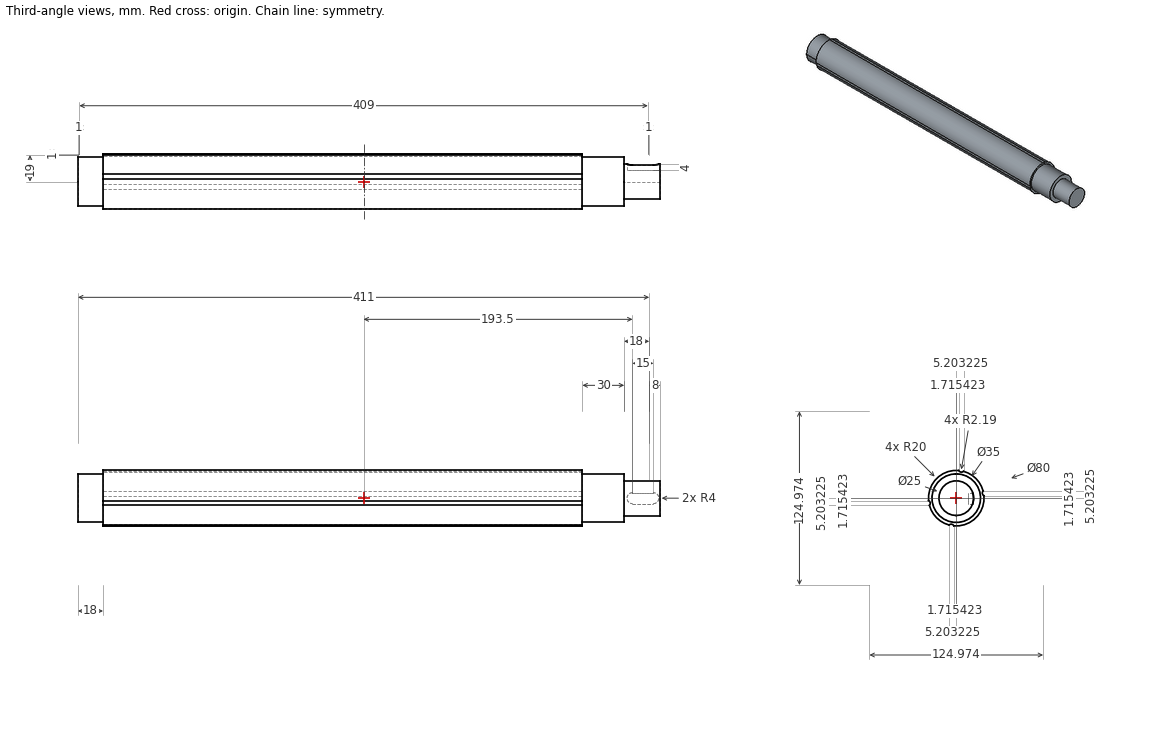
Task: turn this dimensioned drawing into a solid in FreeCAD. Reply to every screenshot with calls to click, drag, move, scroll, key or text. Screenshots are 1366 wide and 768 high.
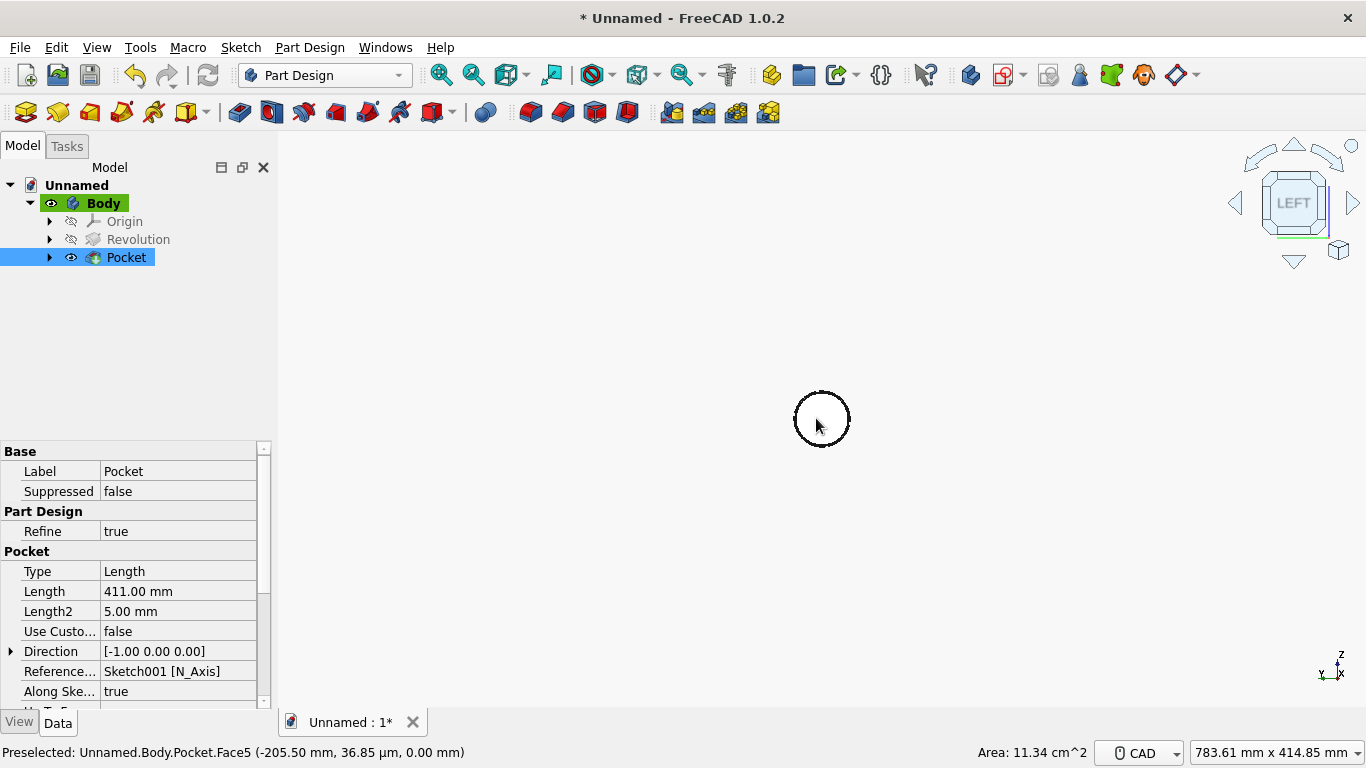
click(1004, 76)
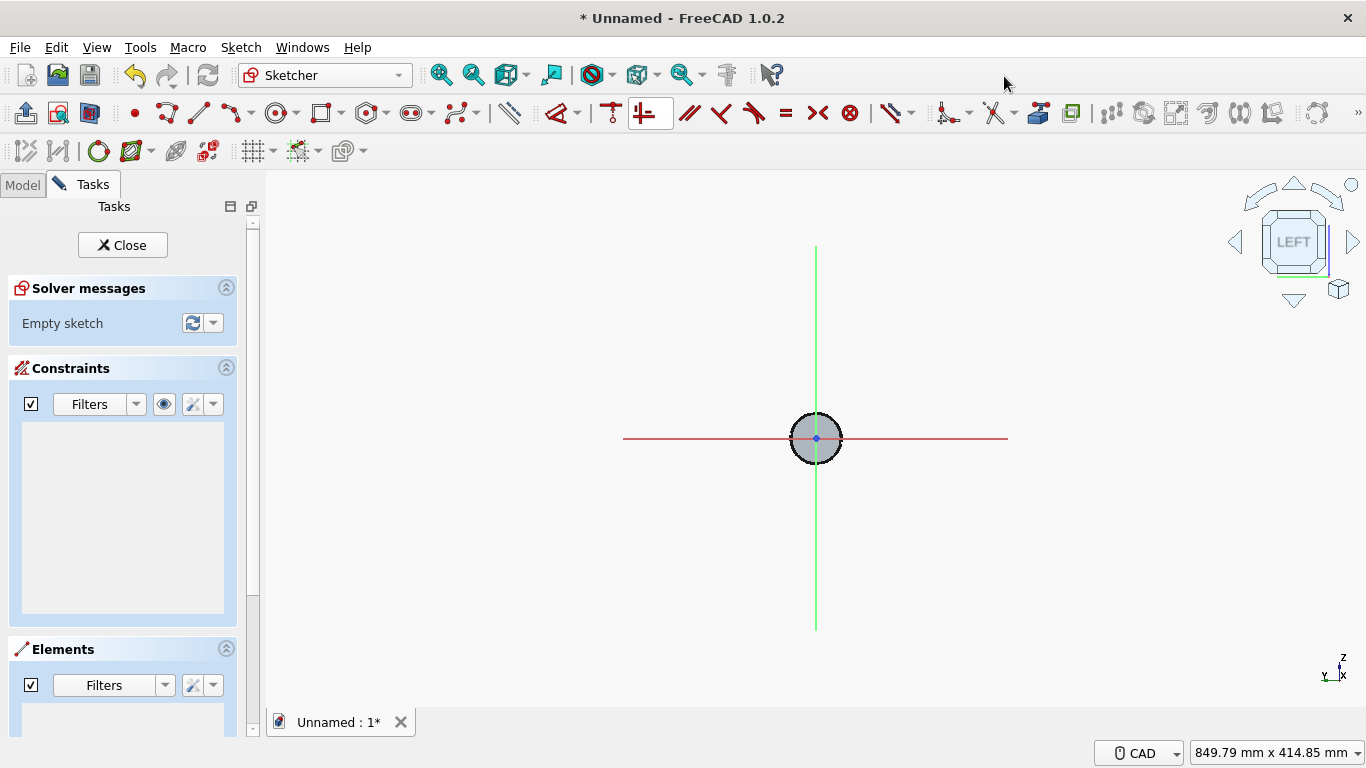
scroll(872, 438, up, 4)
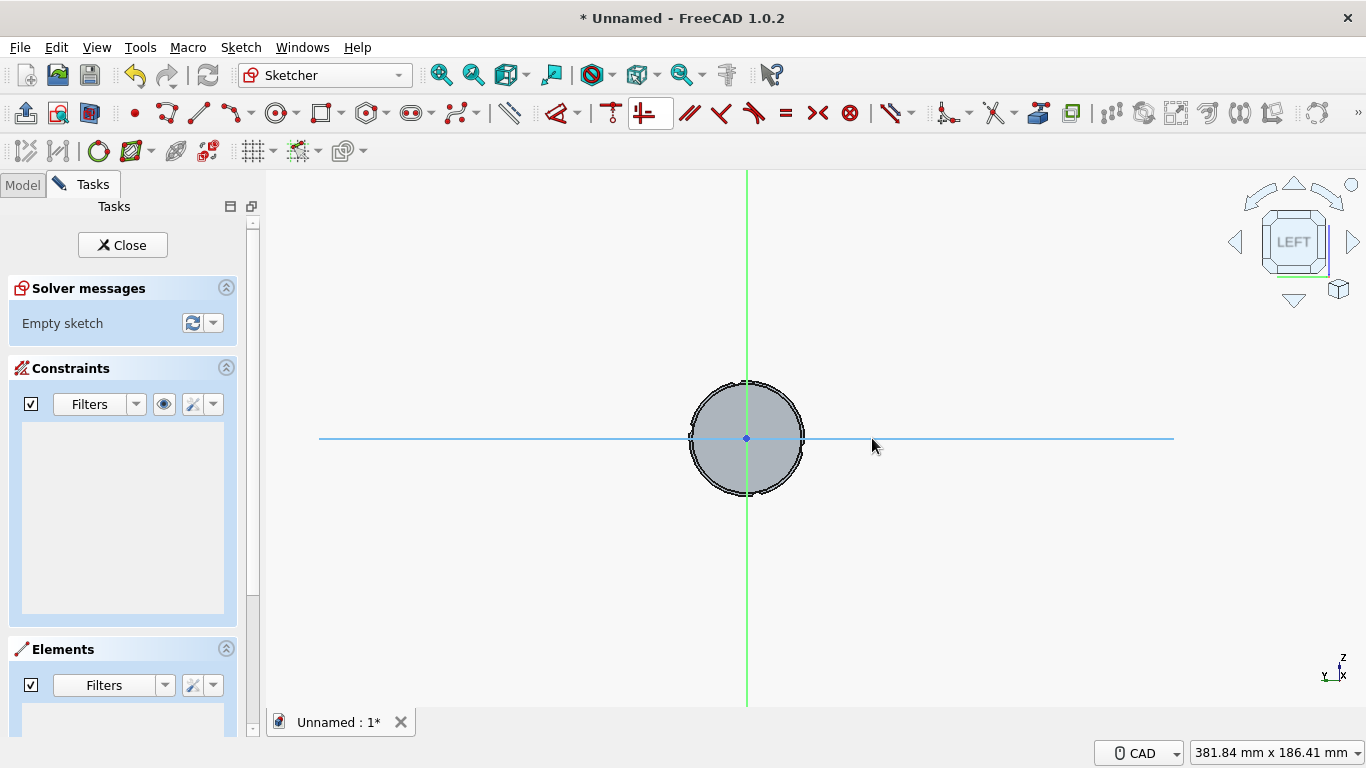
key(g)
key(v)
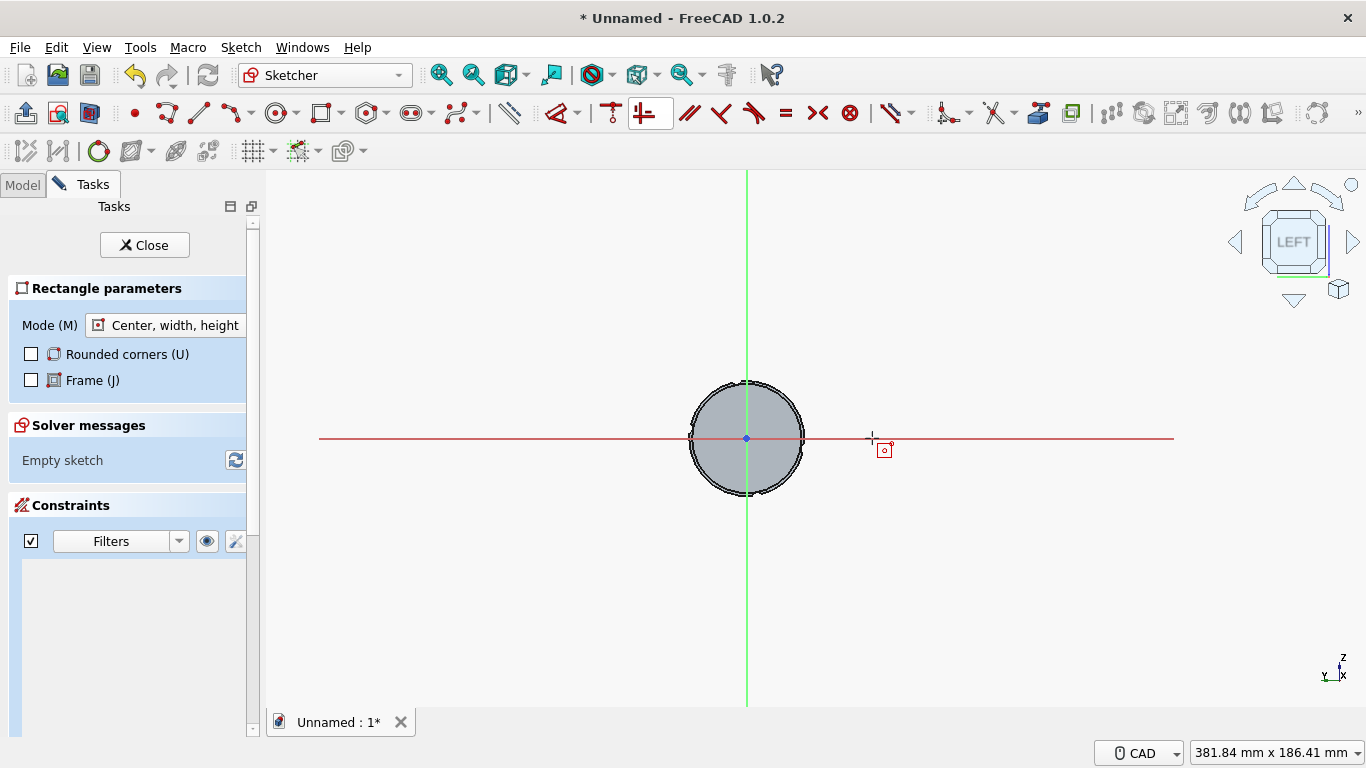
click(747, 438)
click(927, 258)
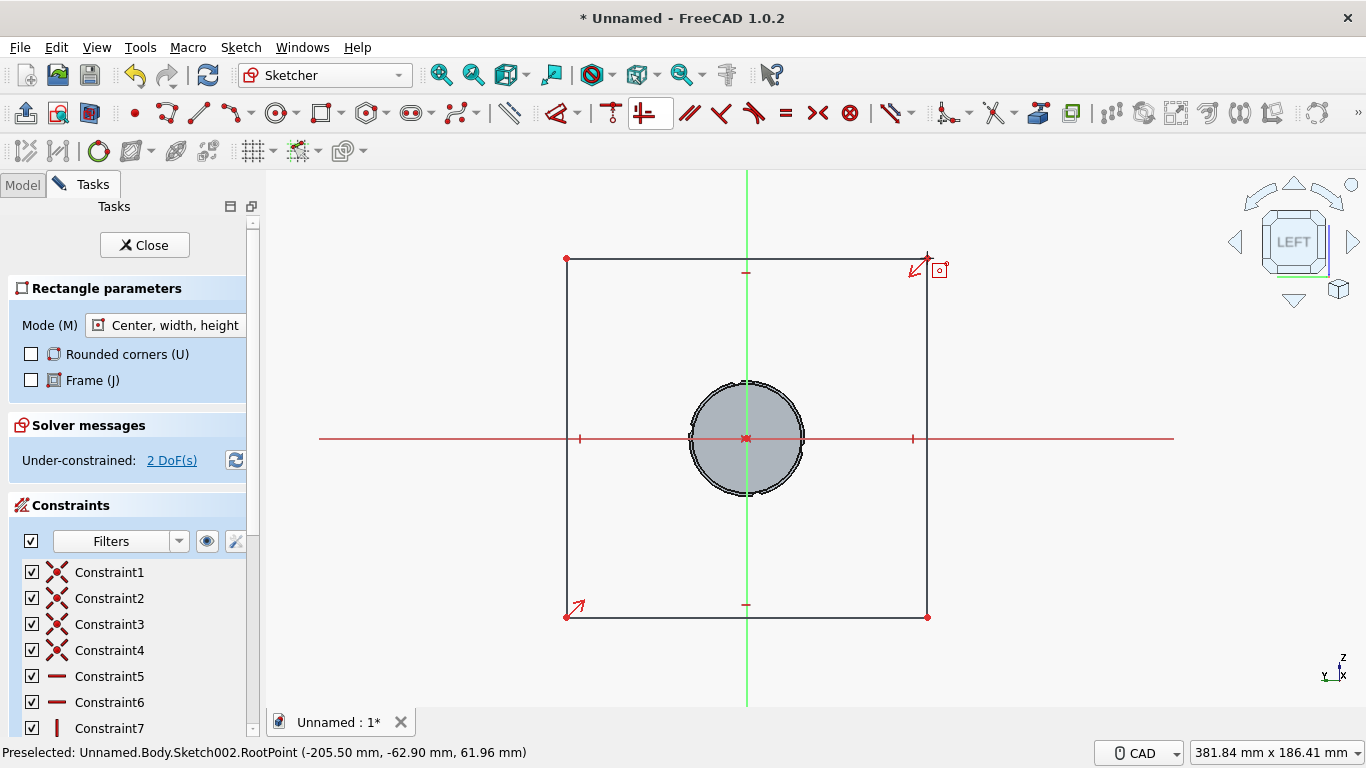
key(g)
key(c)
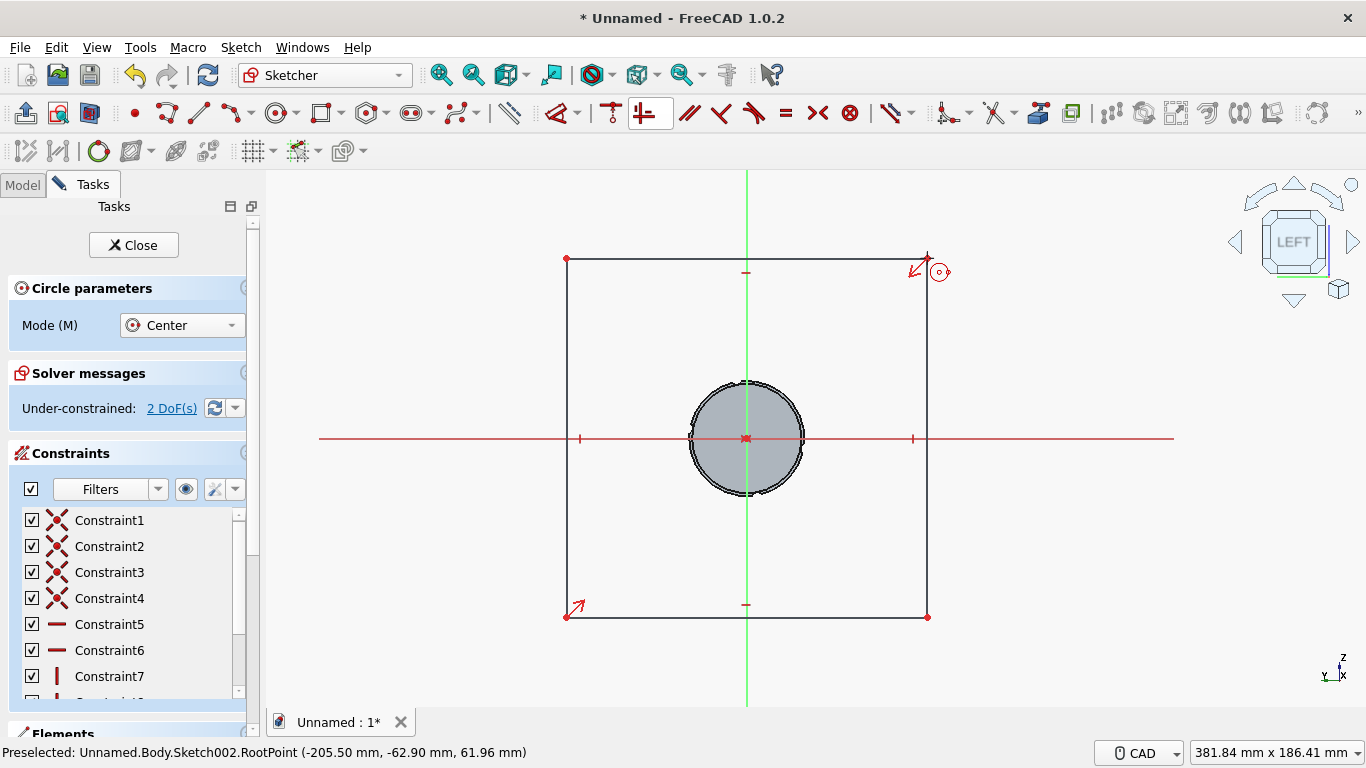
click(747, 438)
click(782, 403)
key(Escape)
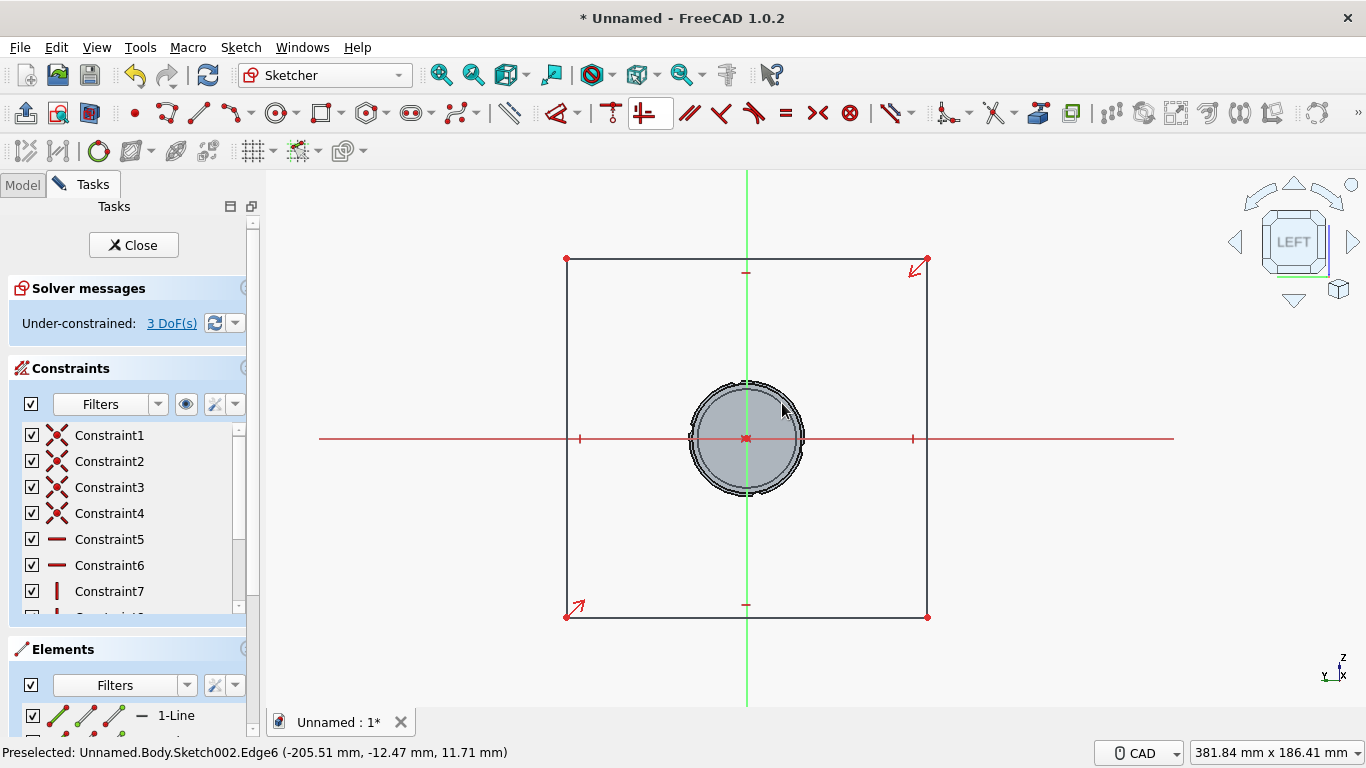
click(556, 114)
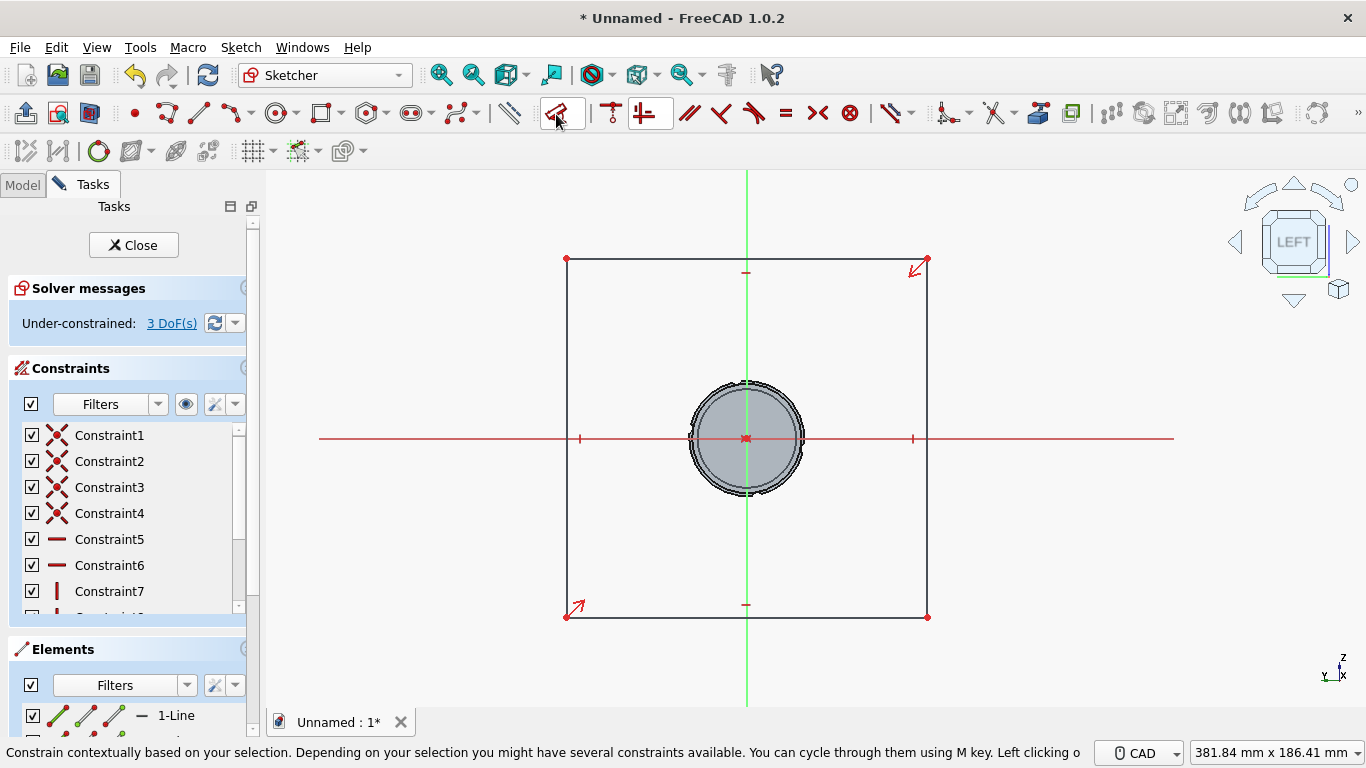
click(782, 404)
click(805, 382)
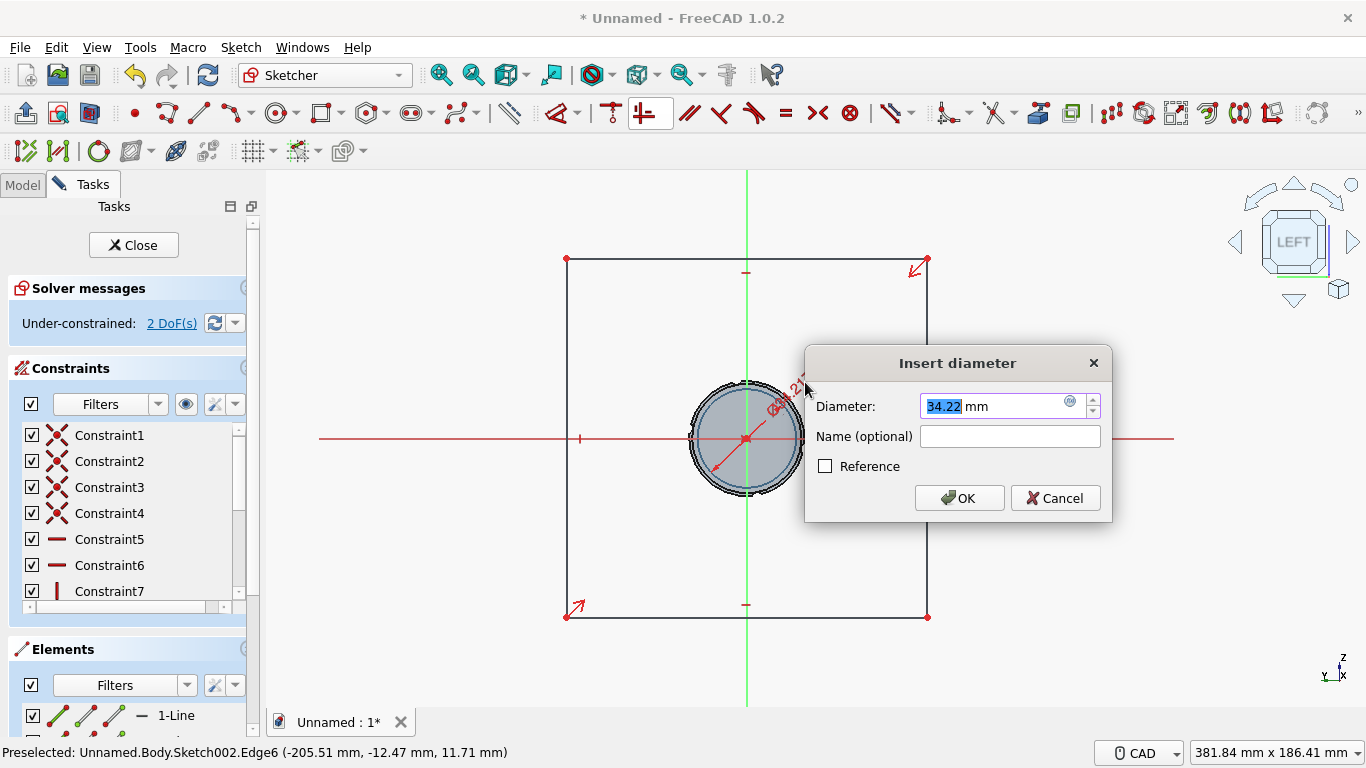
text(35)
key(Return)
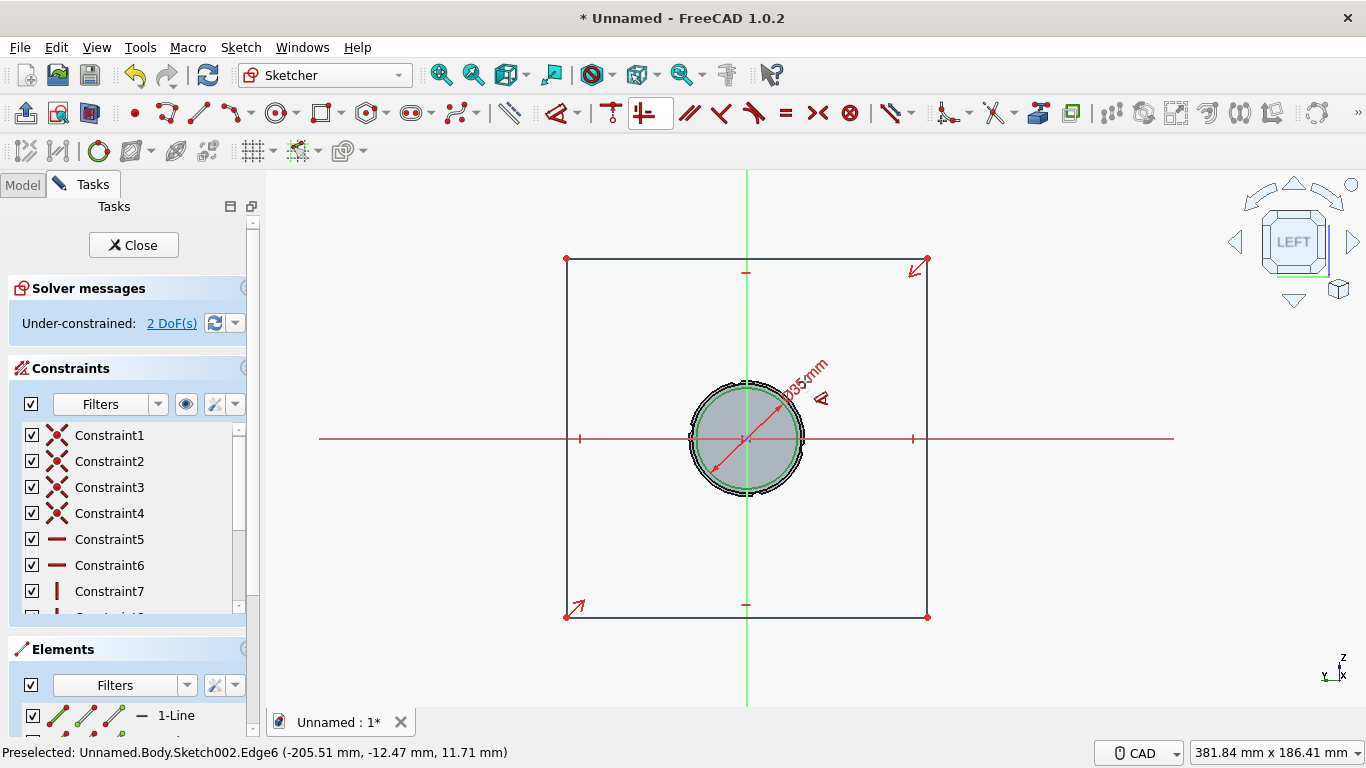
click(675, 618)
click(664, 652)